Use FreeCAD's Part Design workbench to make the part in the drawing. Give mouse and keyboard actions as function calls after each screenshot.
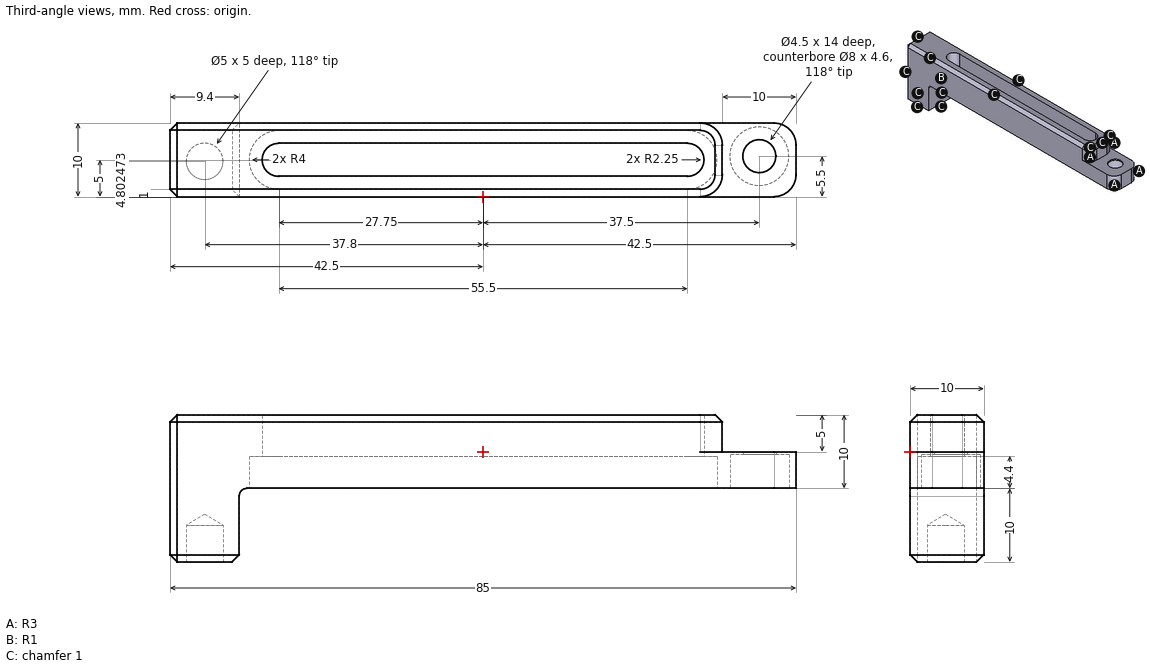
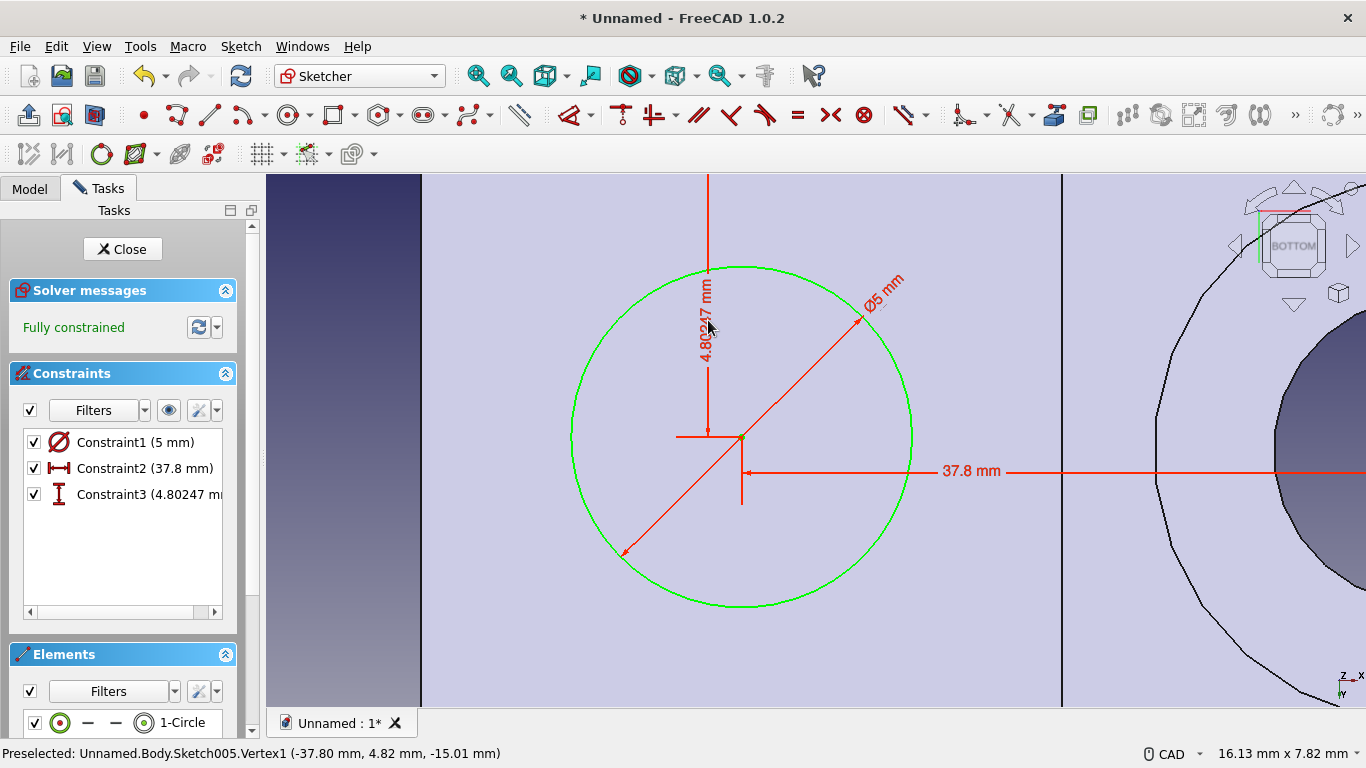
click(123, 249)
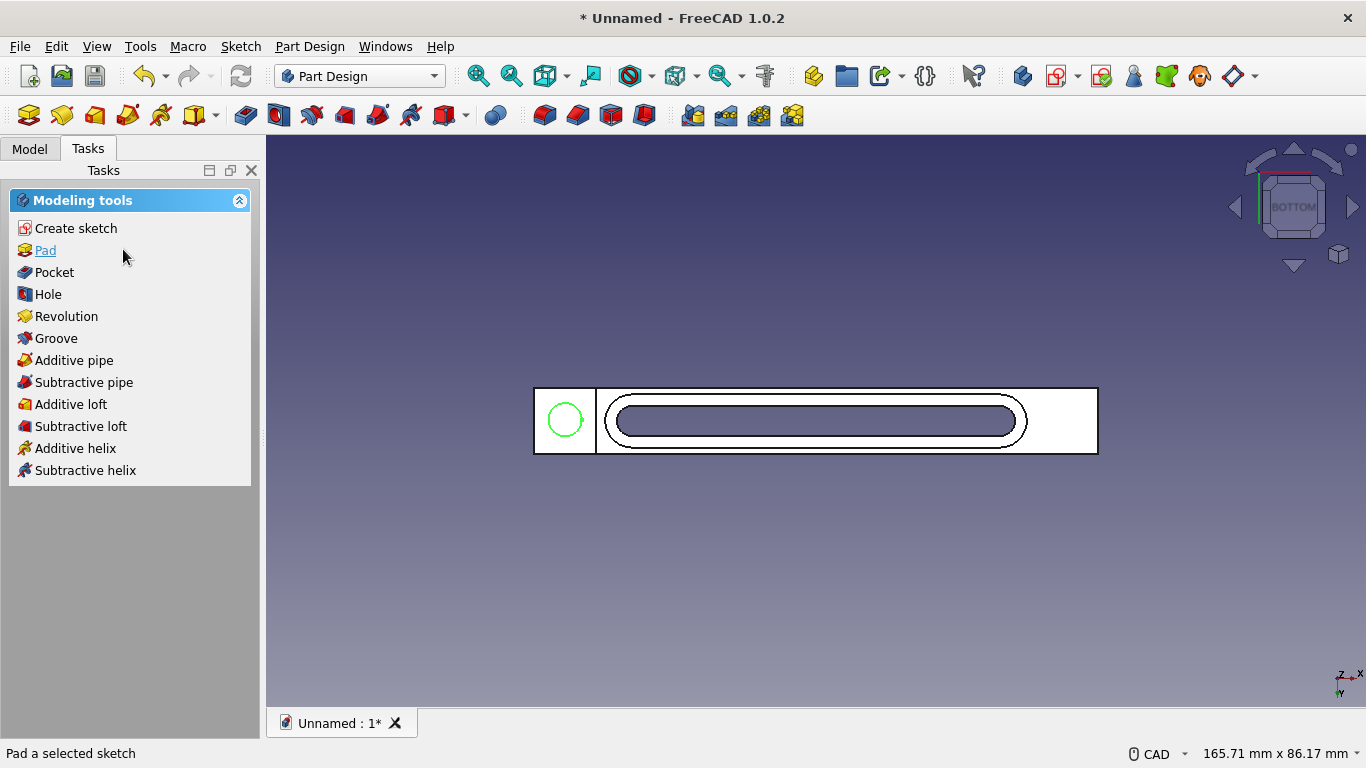
click(279, 116)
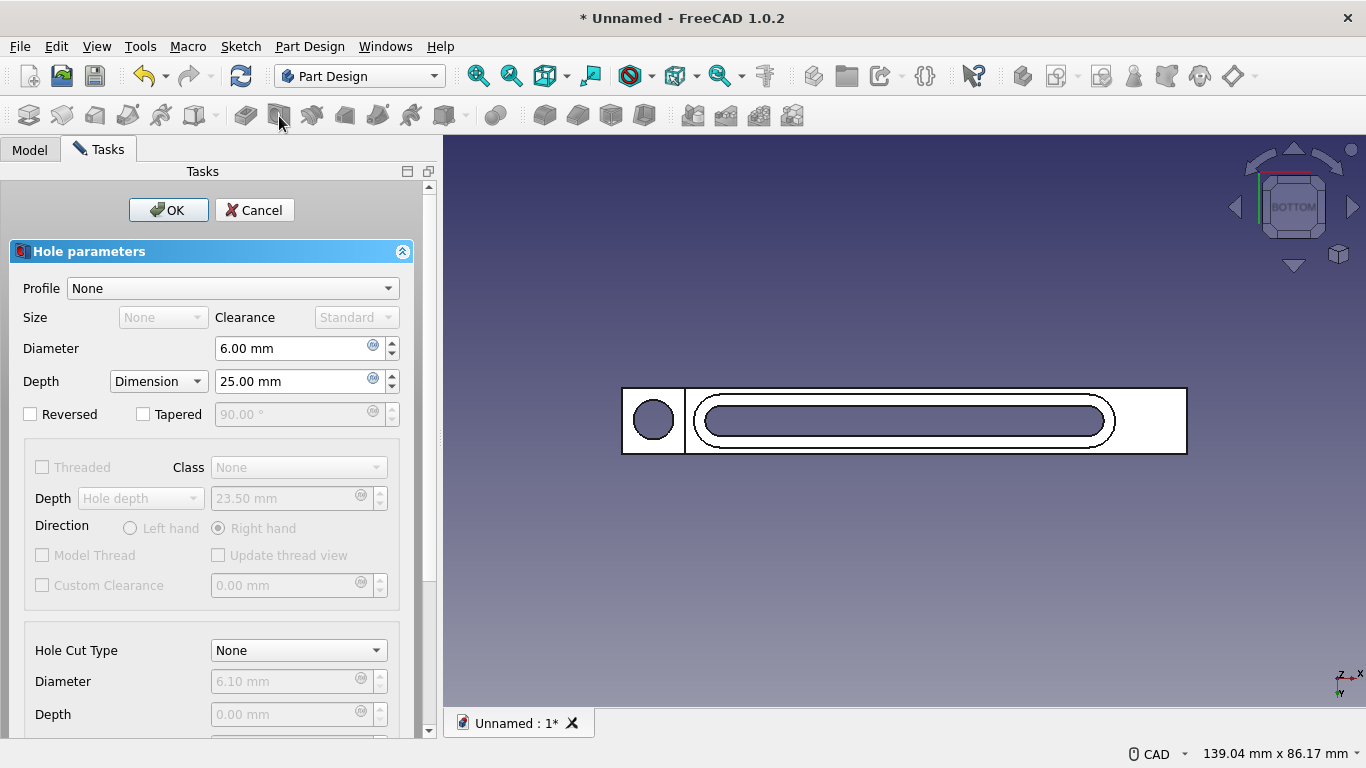
triple_click(300, 348)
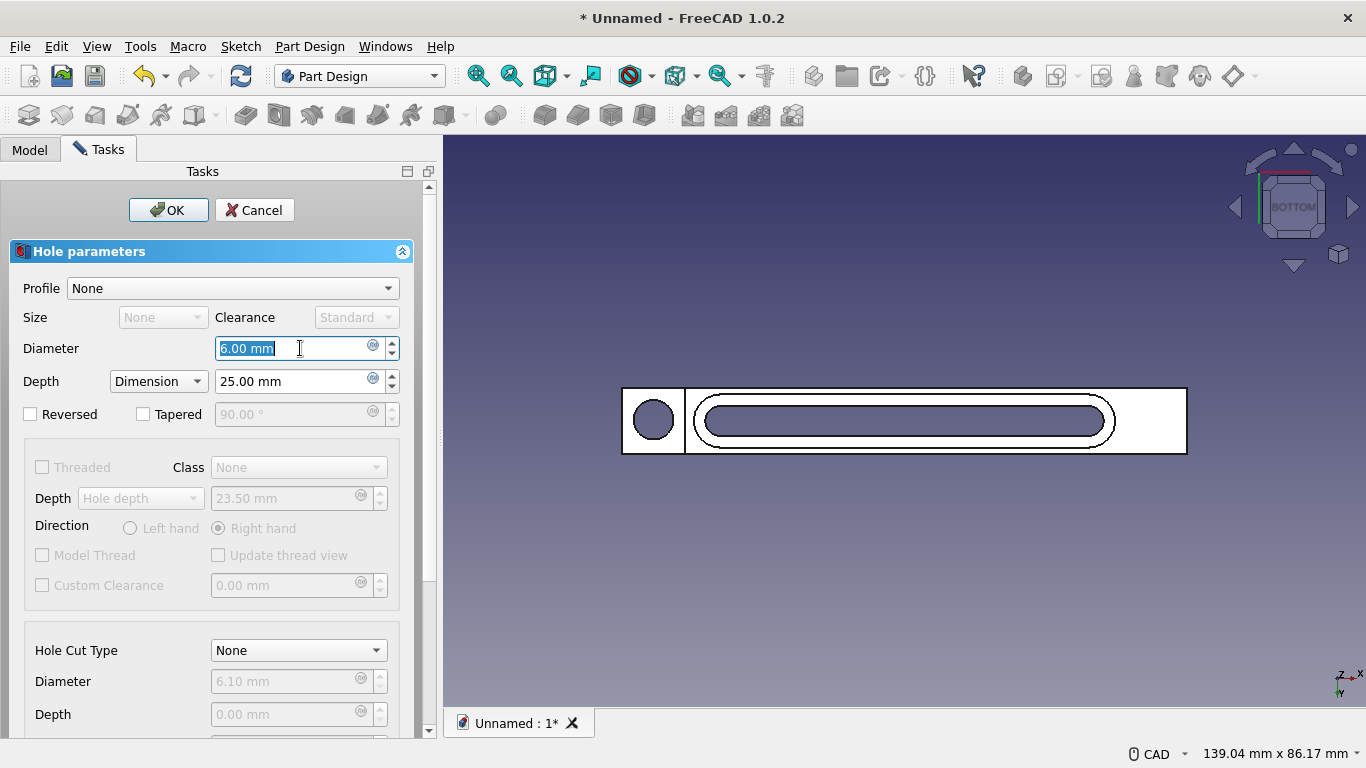
text(5)
key(Tab)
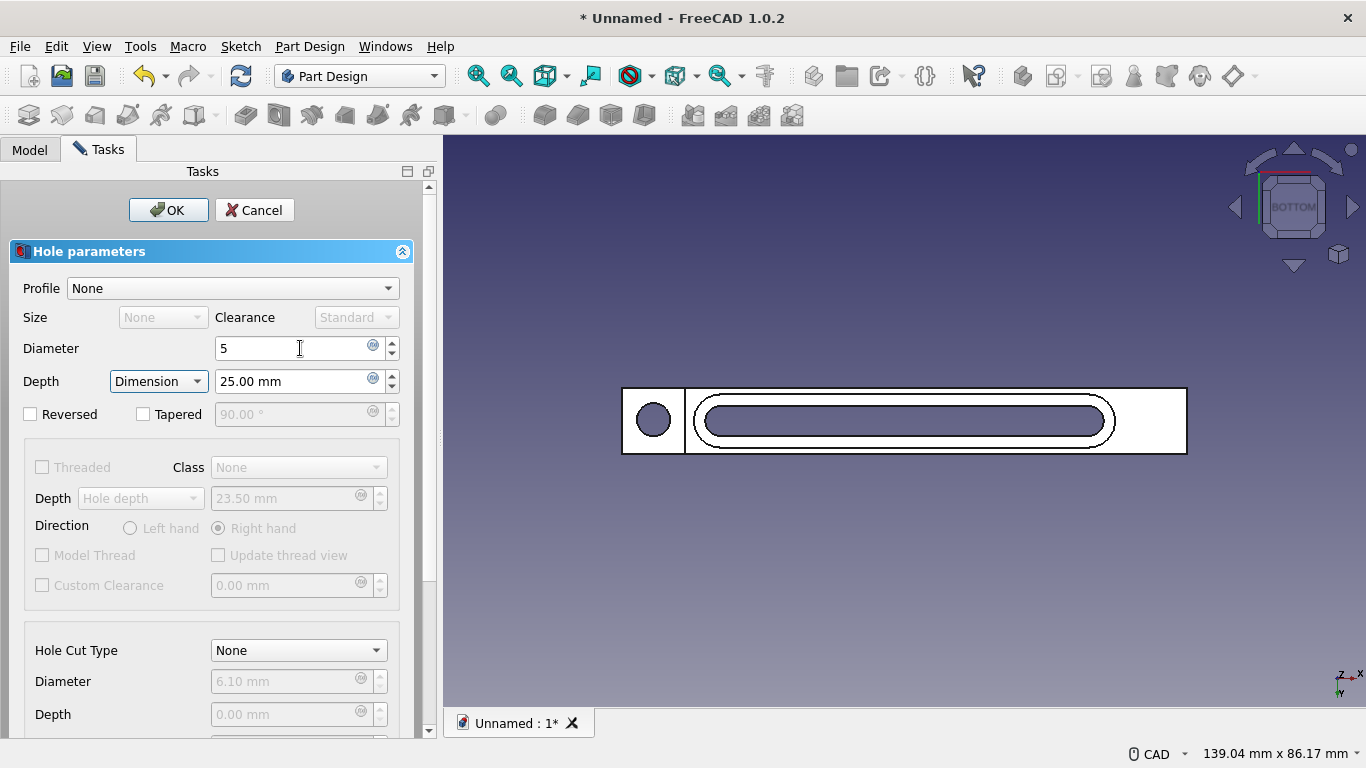
triple_click(300, 382)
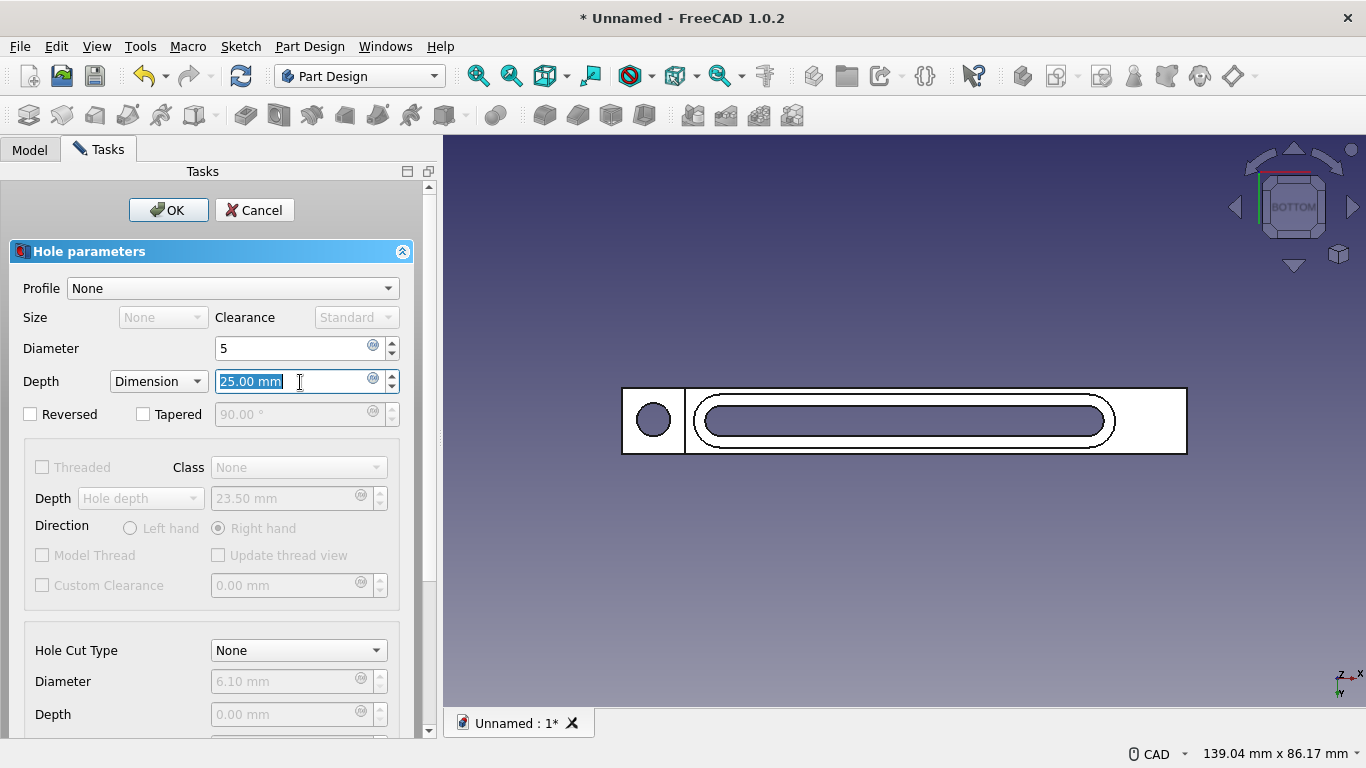
text(5)
key(Tab)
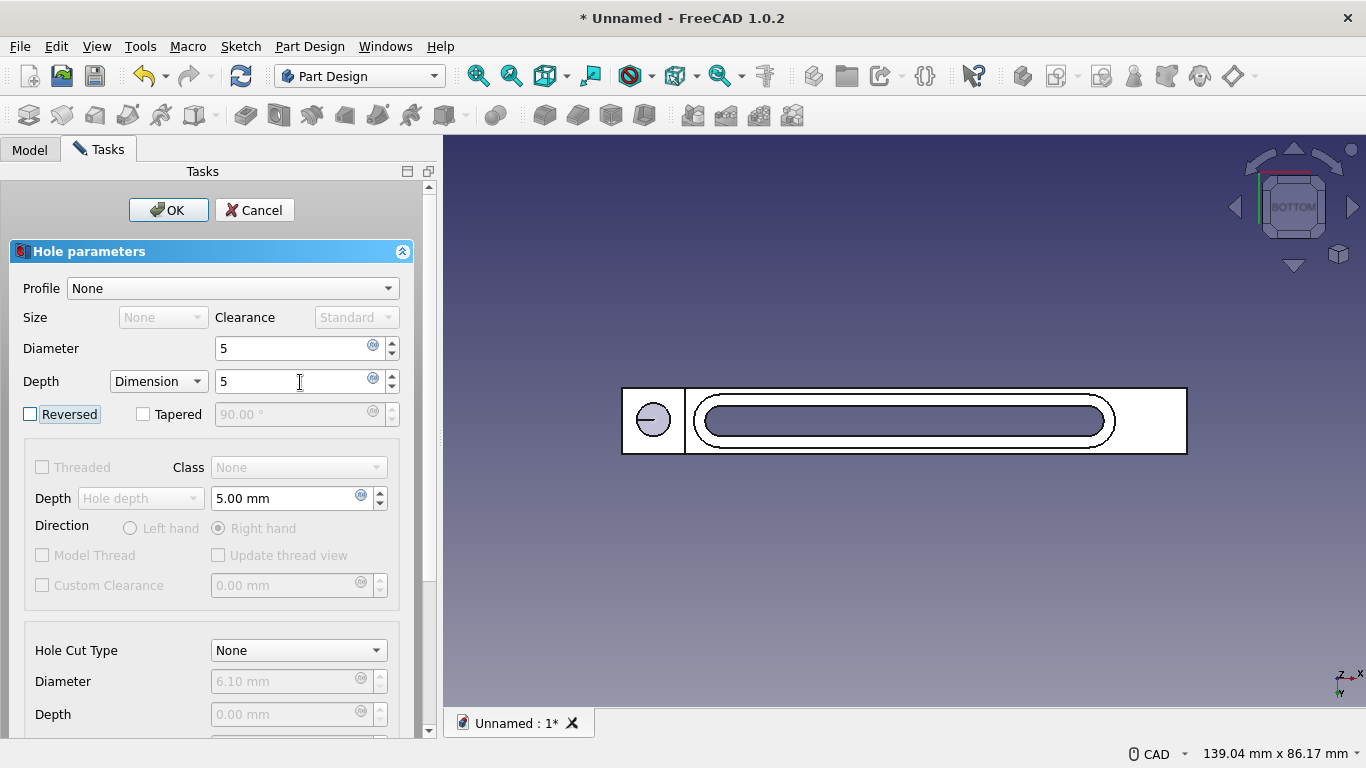
click(169, 210)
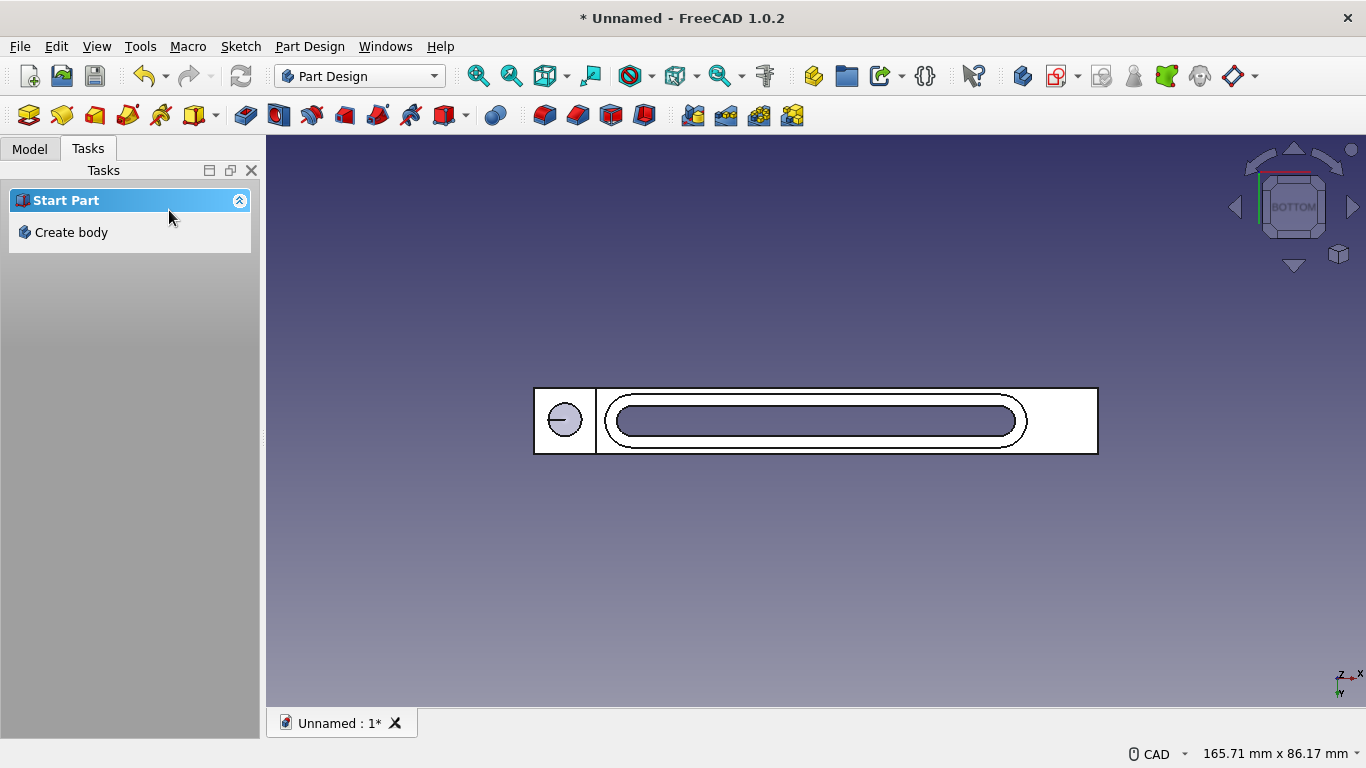
click(1062, 420)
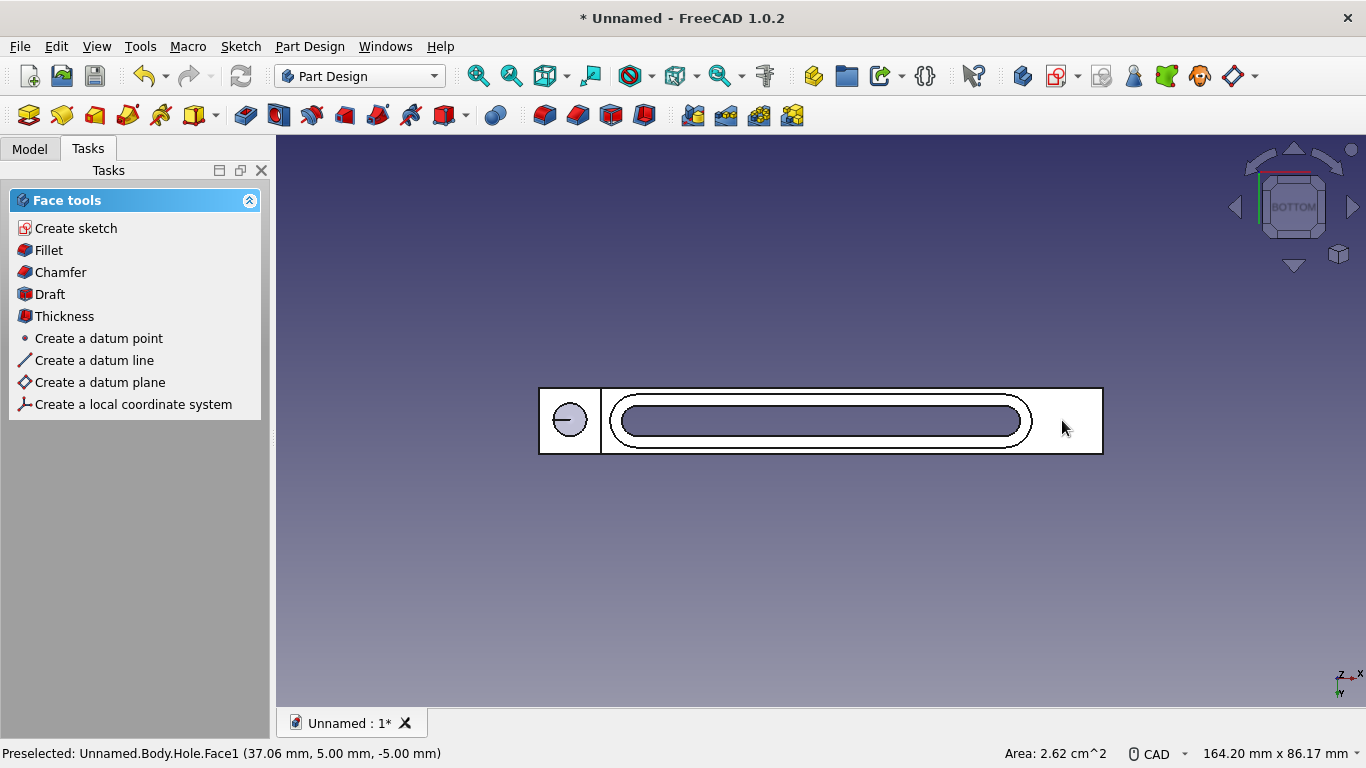
click(1056, 76)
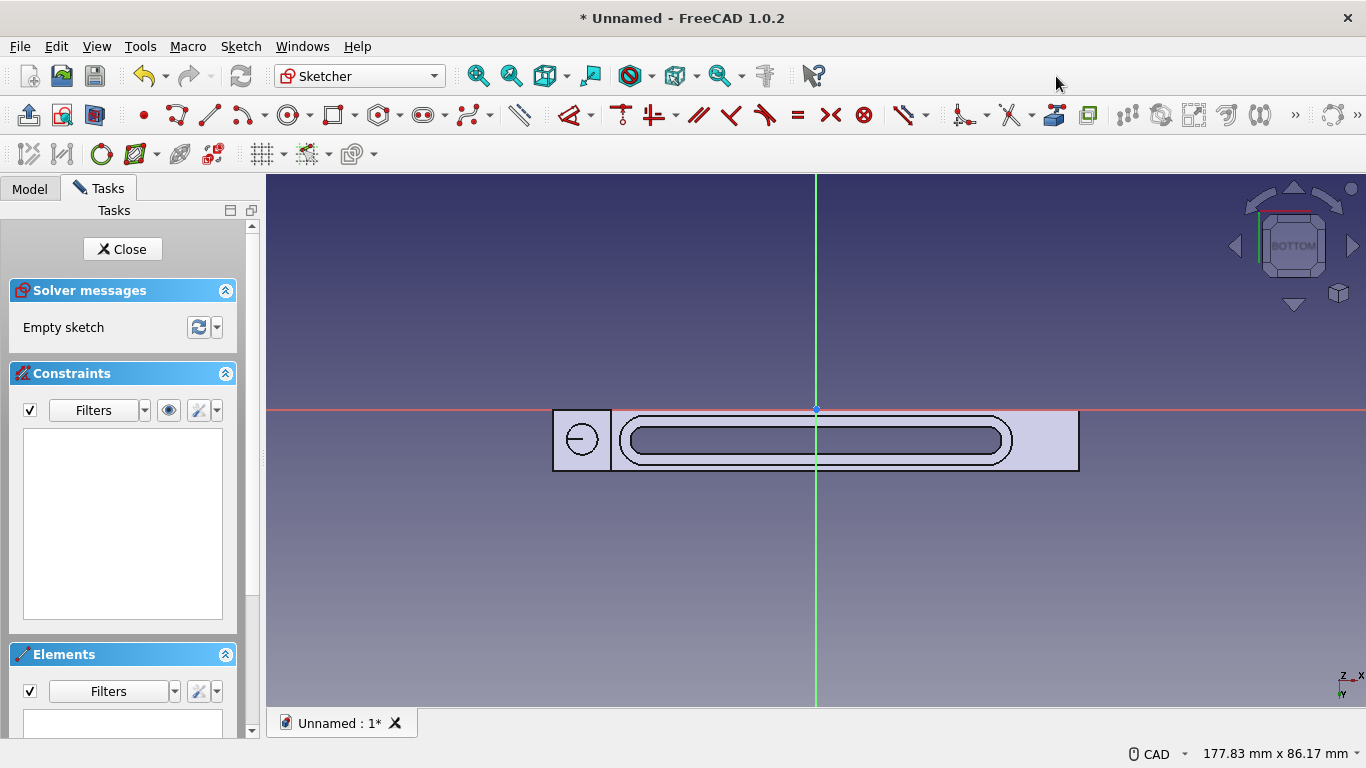
scroll(1078, 444, up, 12)